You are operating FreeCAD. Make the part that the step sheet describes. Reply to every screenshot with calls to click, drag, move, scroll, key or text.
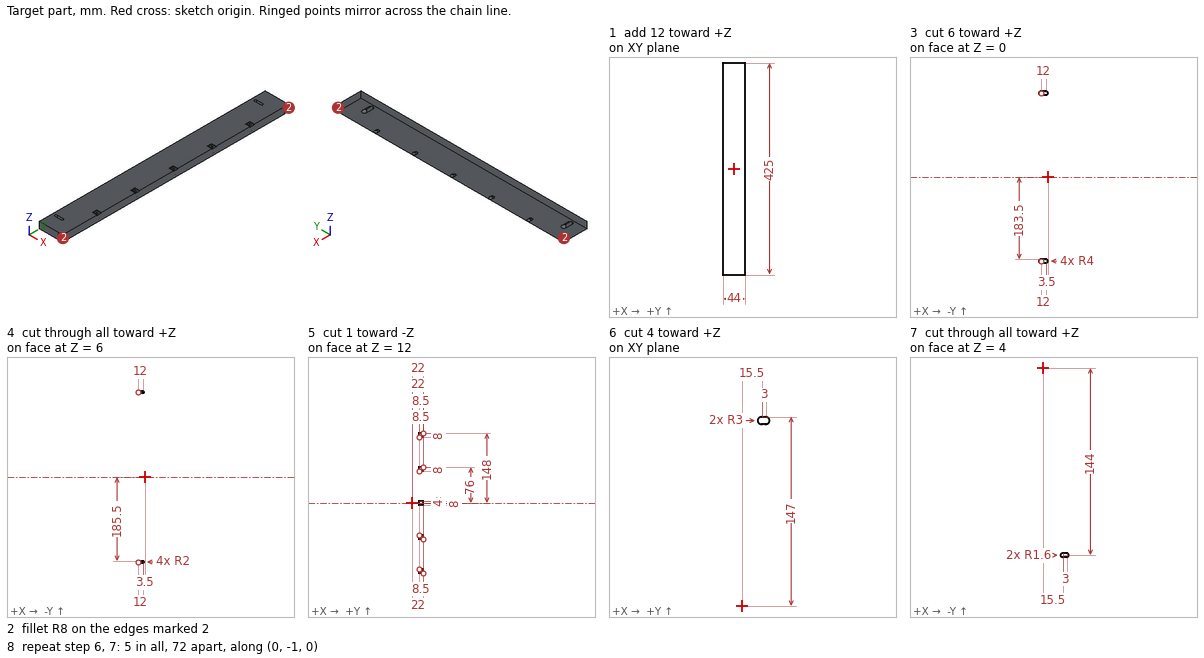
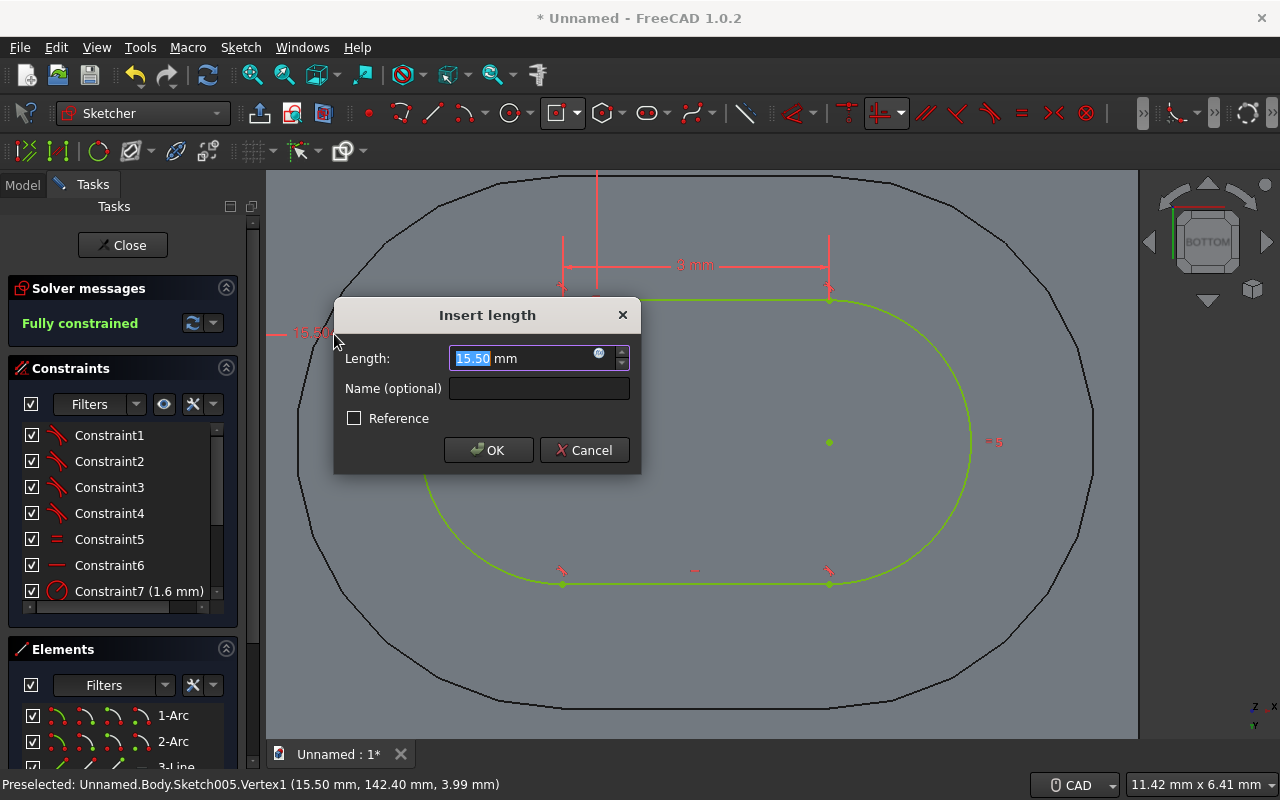
text(15.5)
key(Return)
key(Escape)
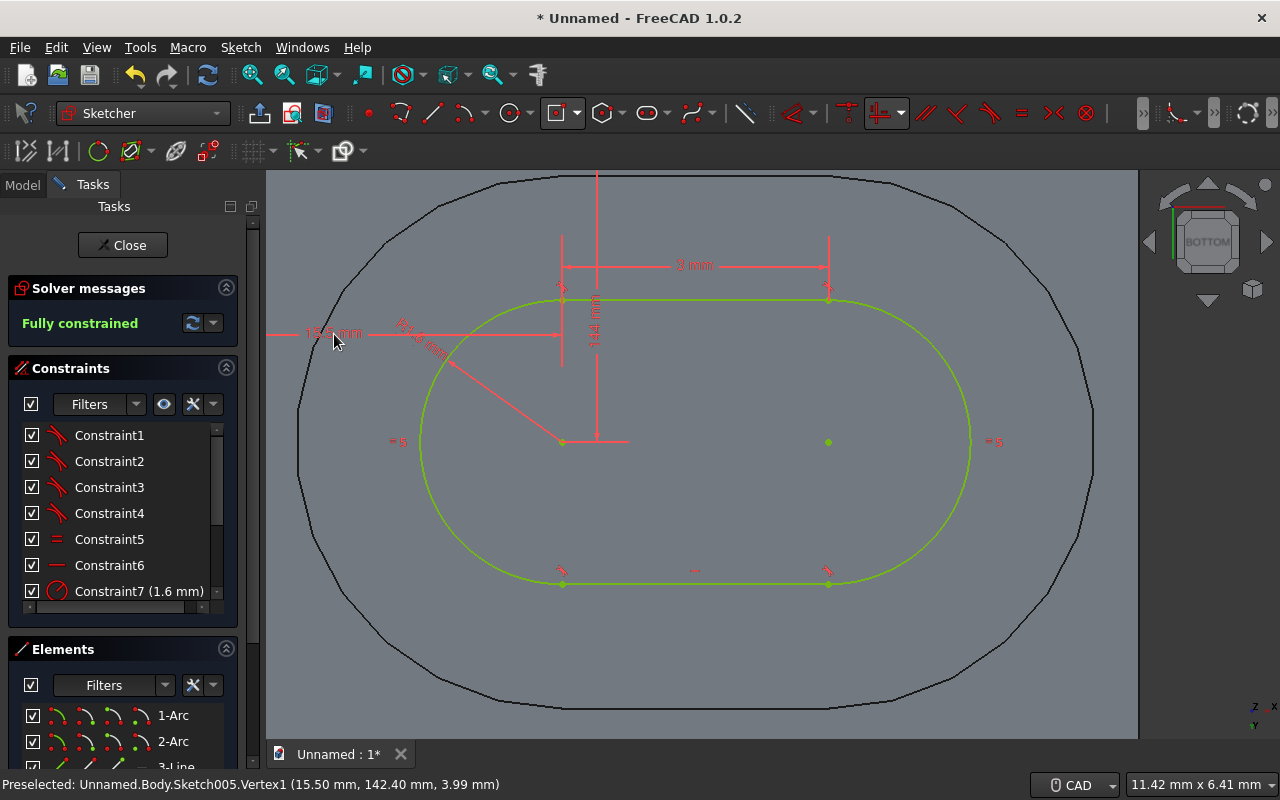
click(123, 245)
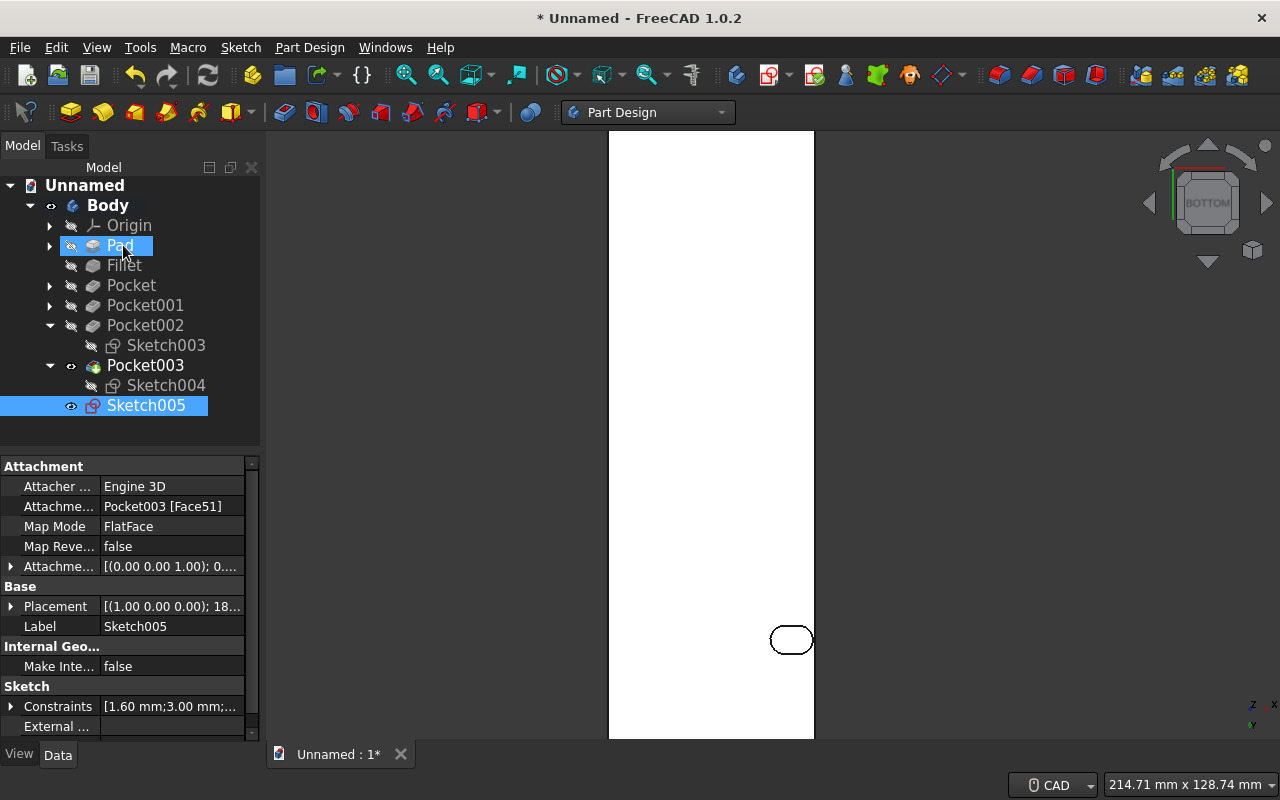
click(286, 112)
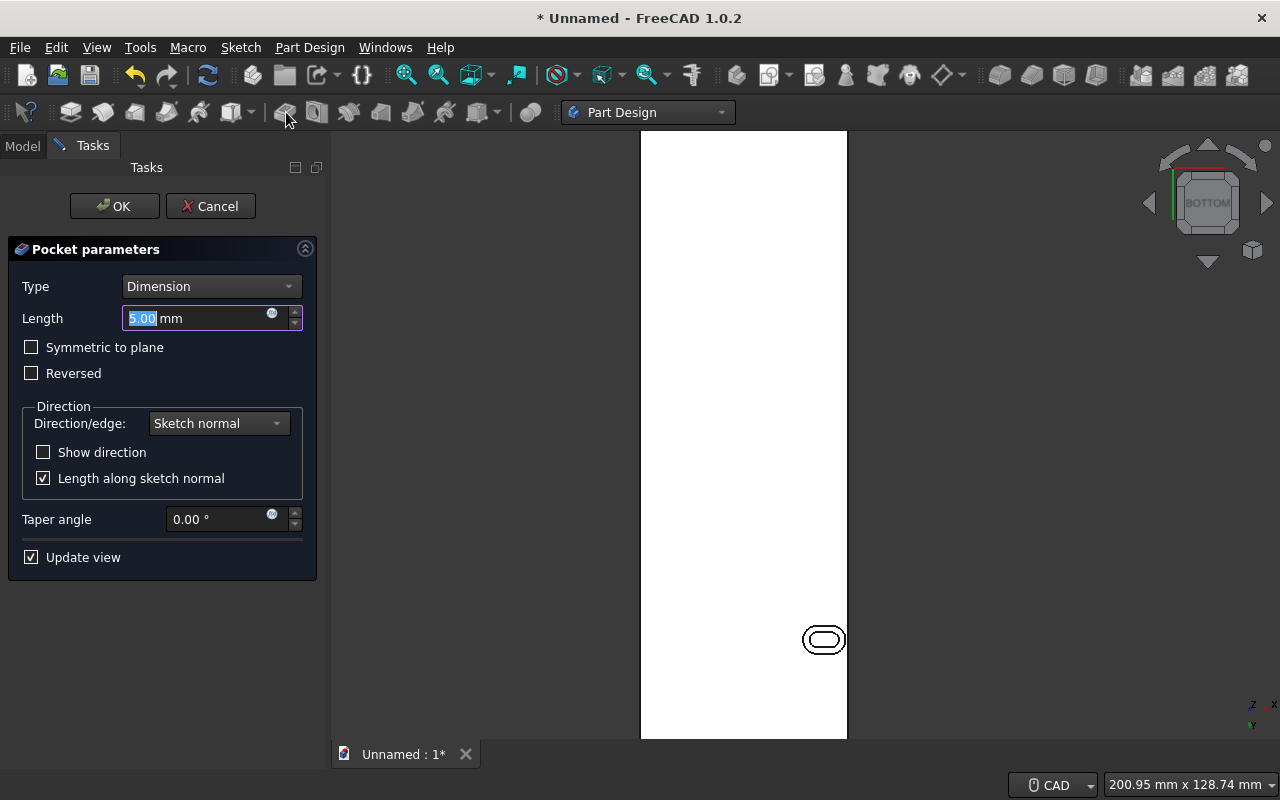
click(212, 286)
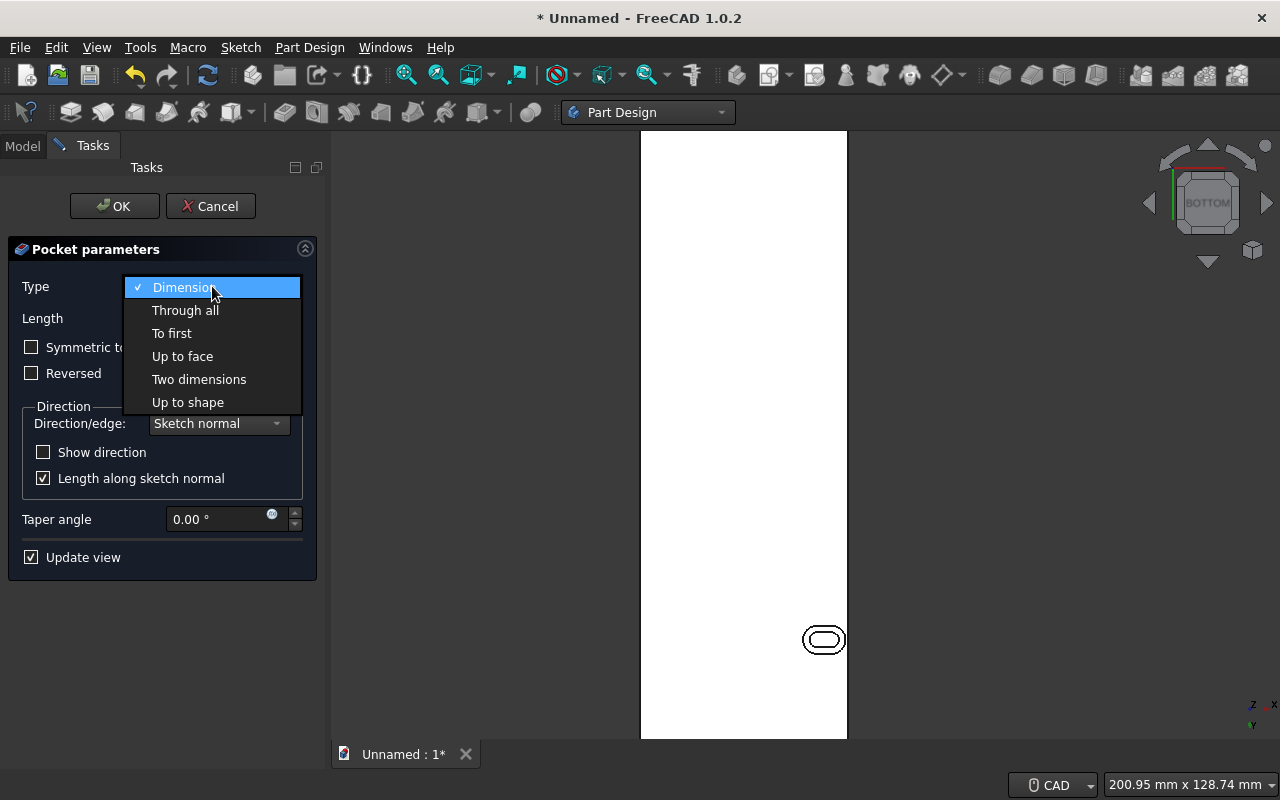
click(212, 310)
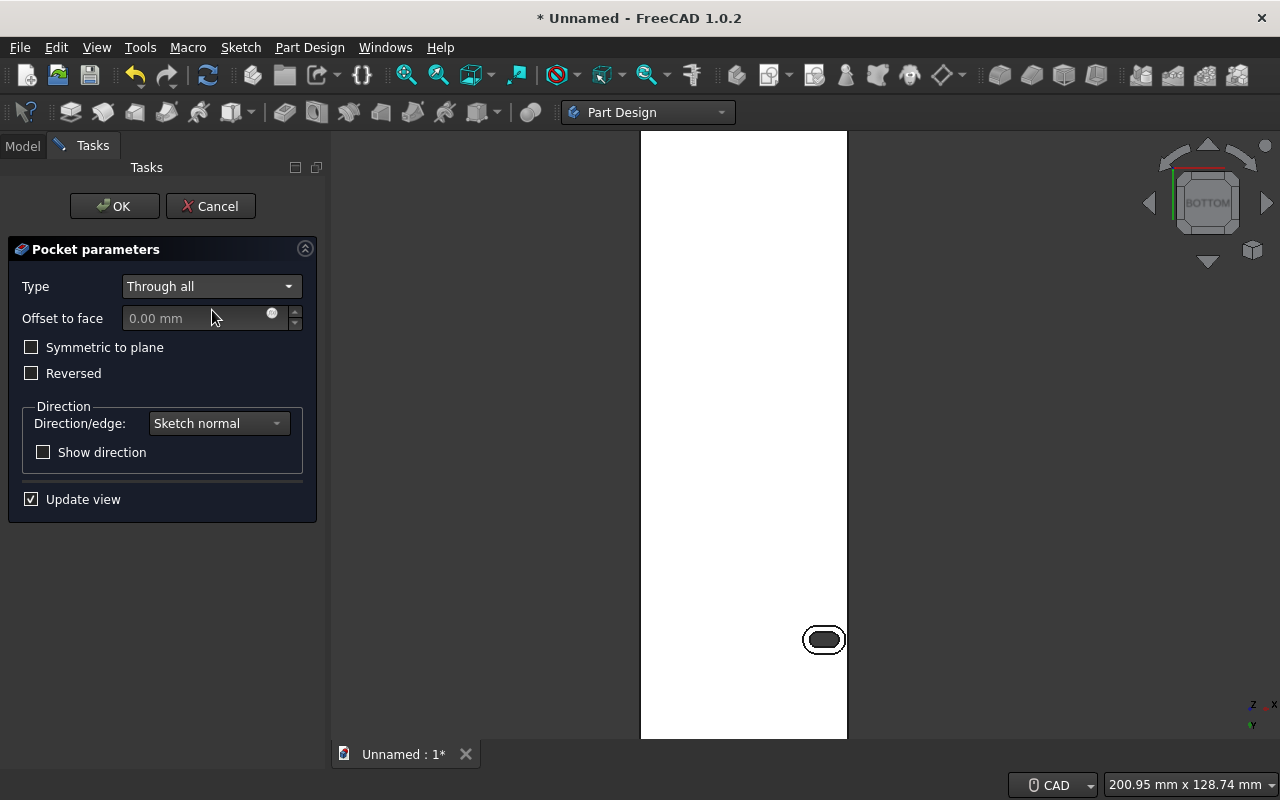
click(115, 206)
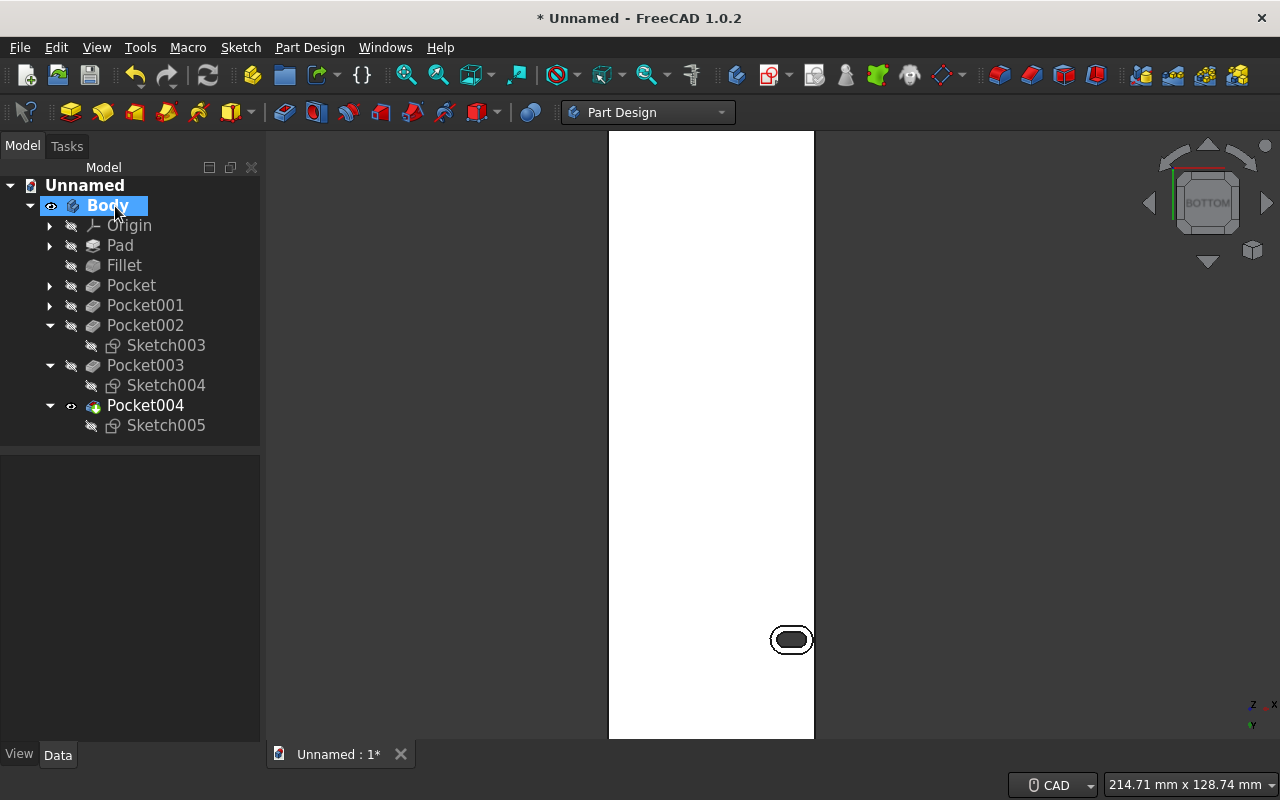
click(408, 76)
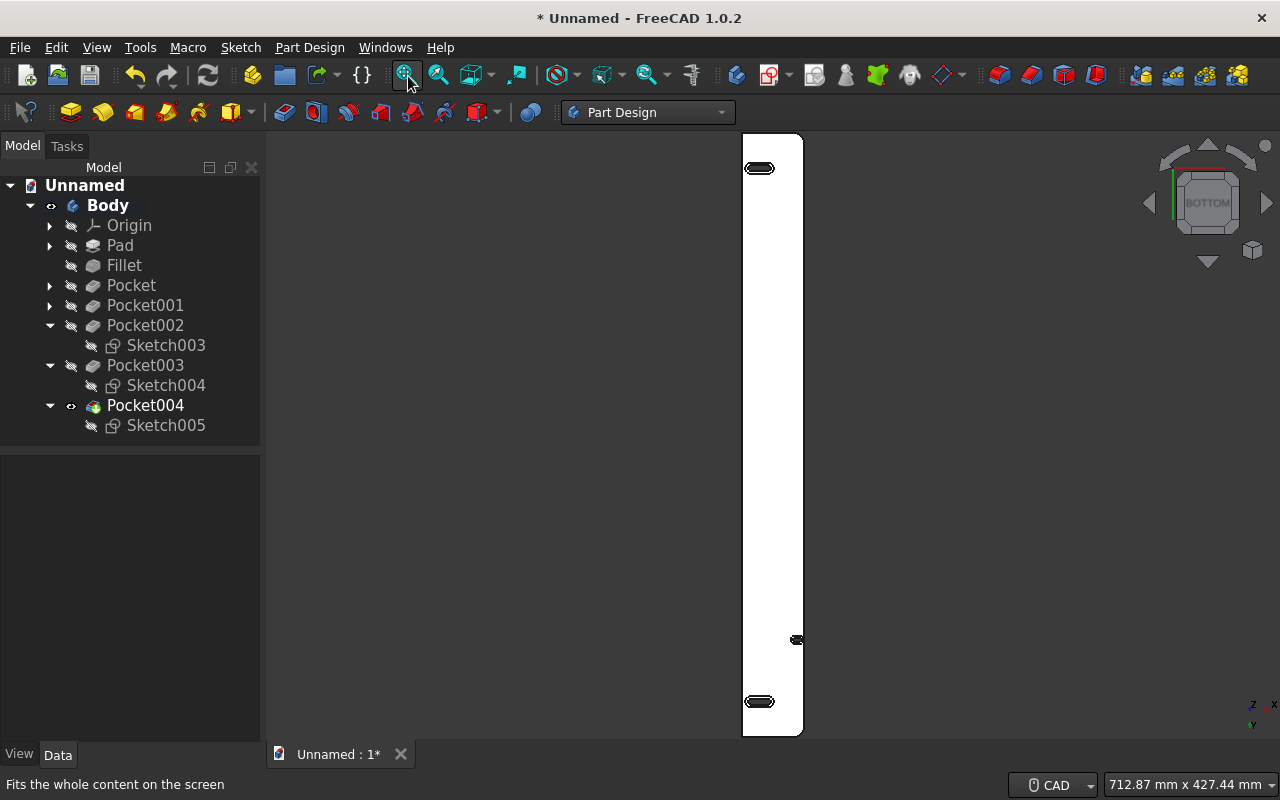
click(116, 366)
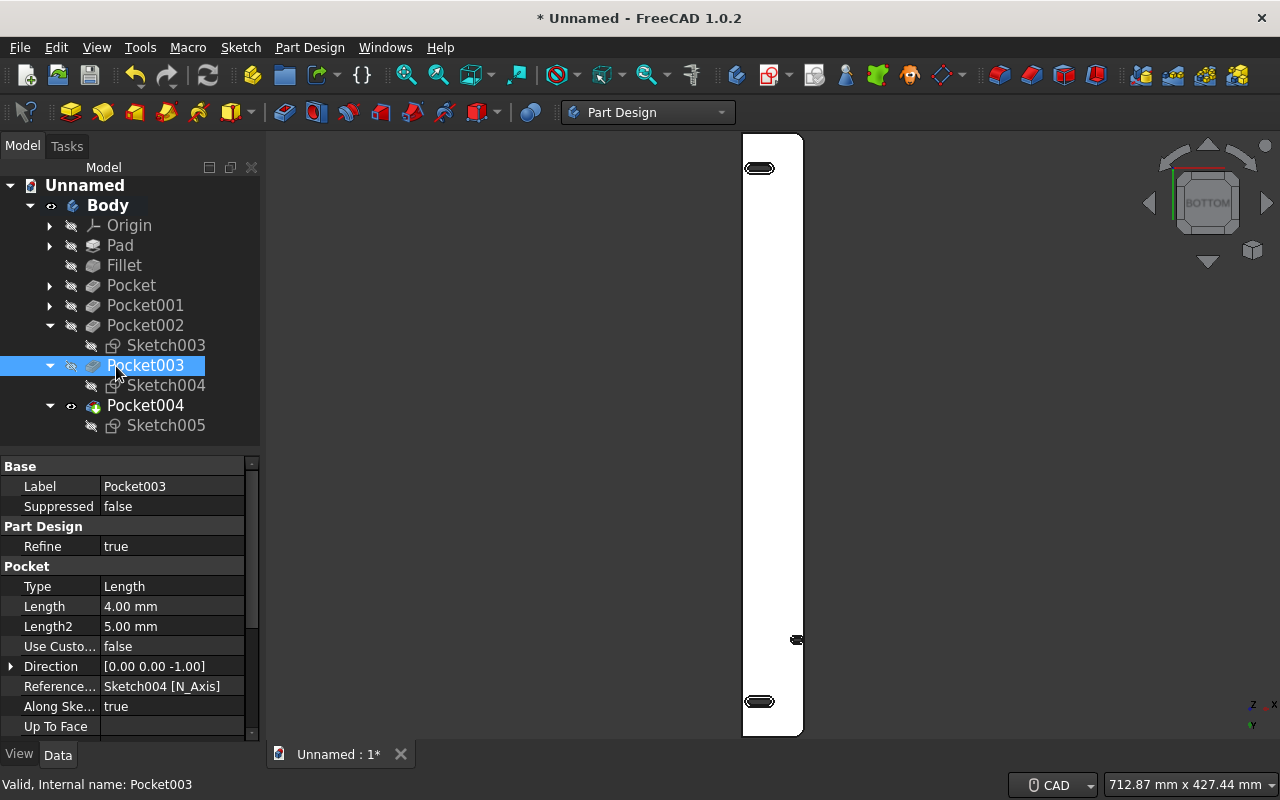
click(116, 406, ctrl)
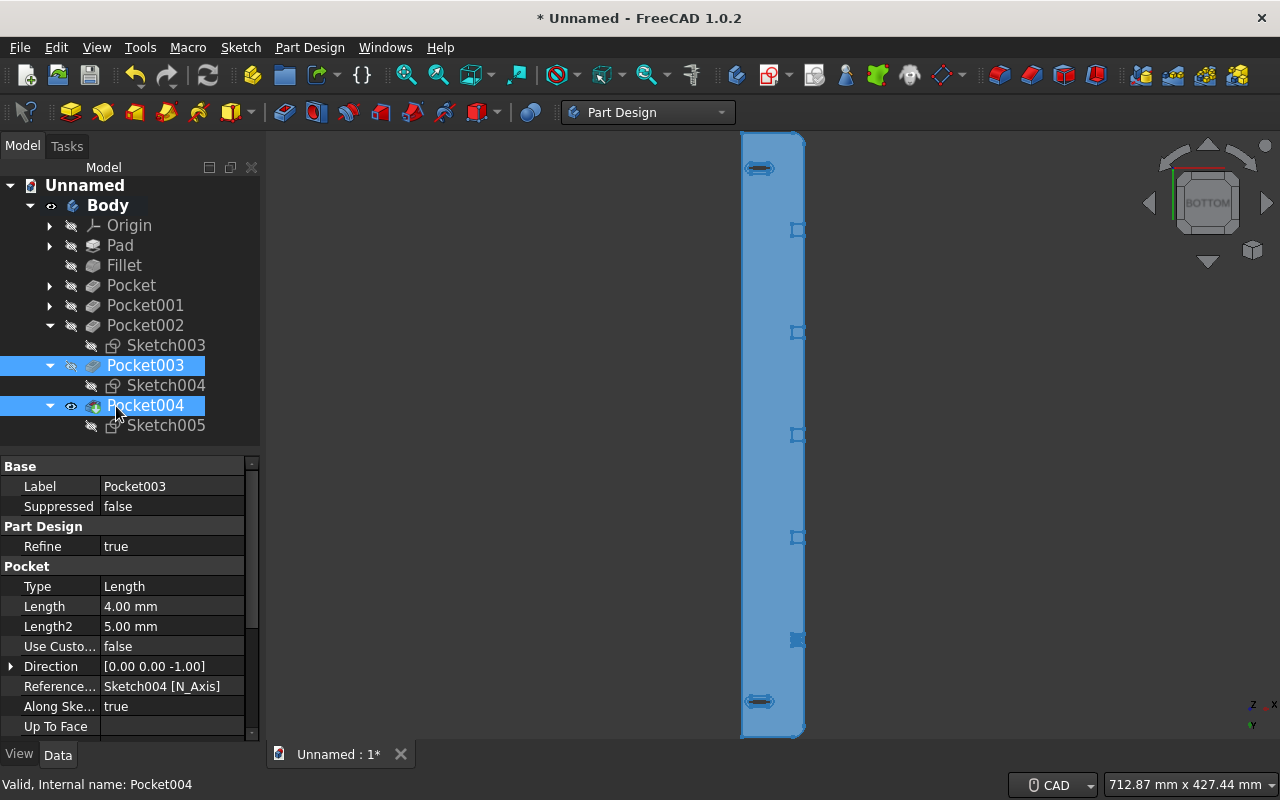
click(1174, 76)